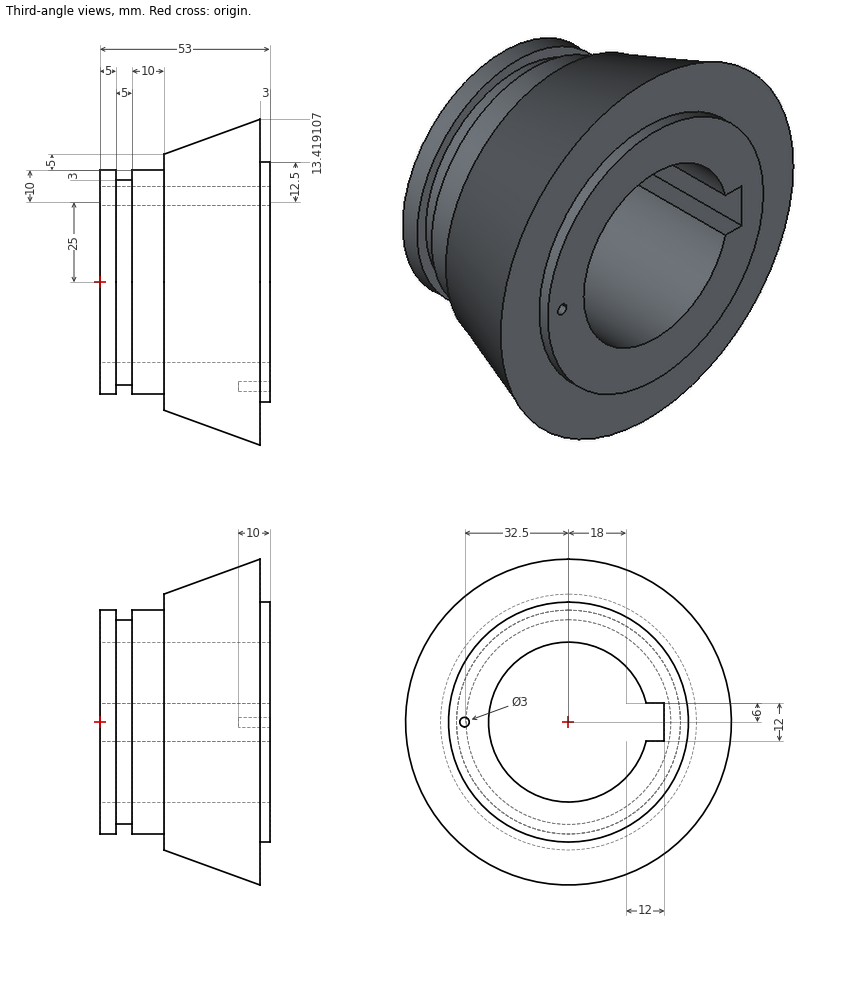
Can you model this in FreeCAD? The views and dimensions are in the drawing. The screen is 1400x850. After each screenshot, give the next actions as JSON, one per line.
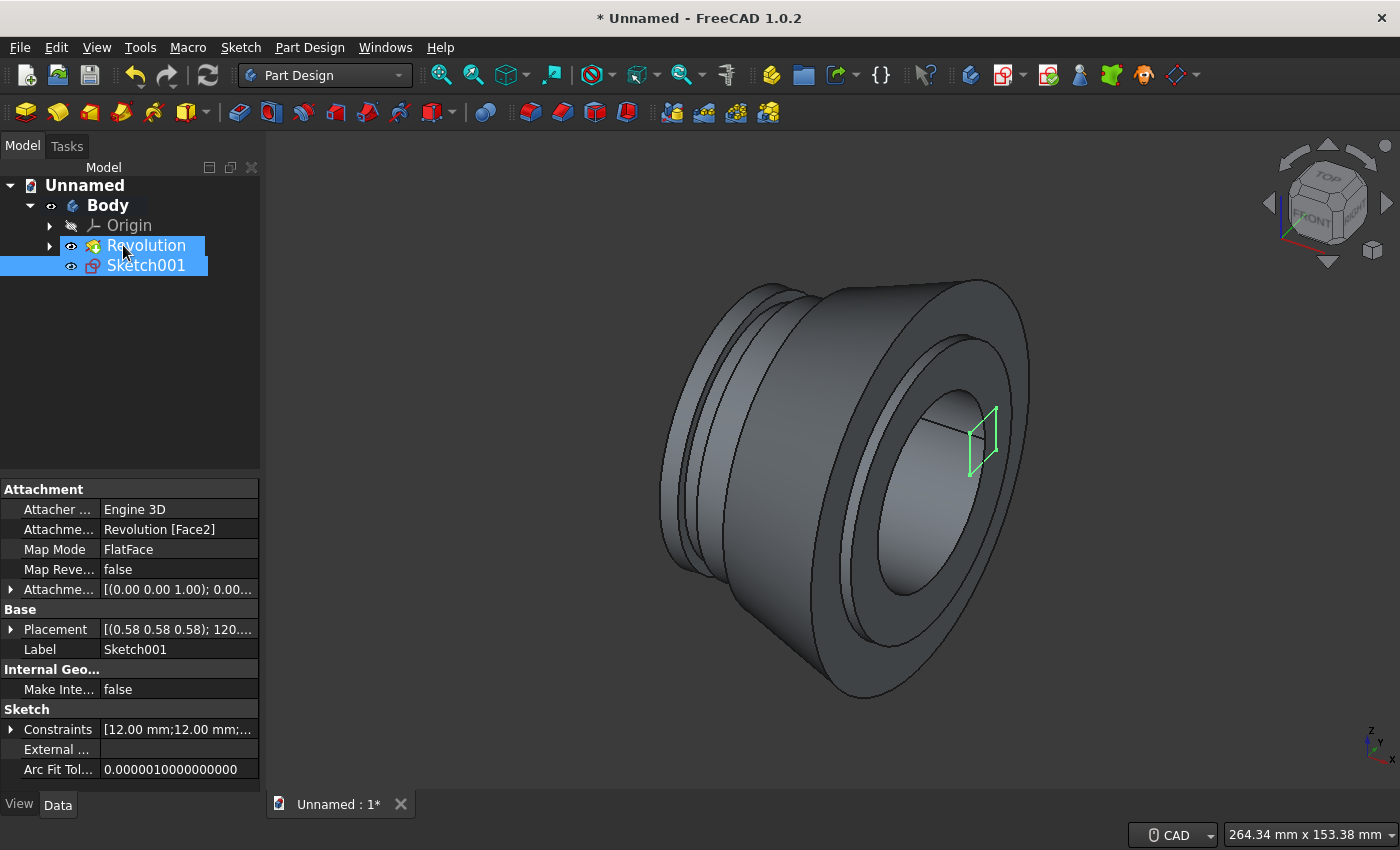
{"action": "left_click", "coordinate": [240, 112]}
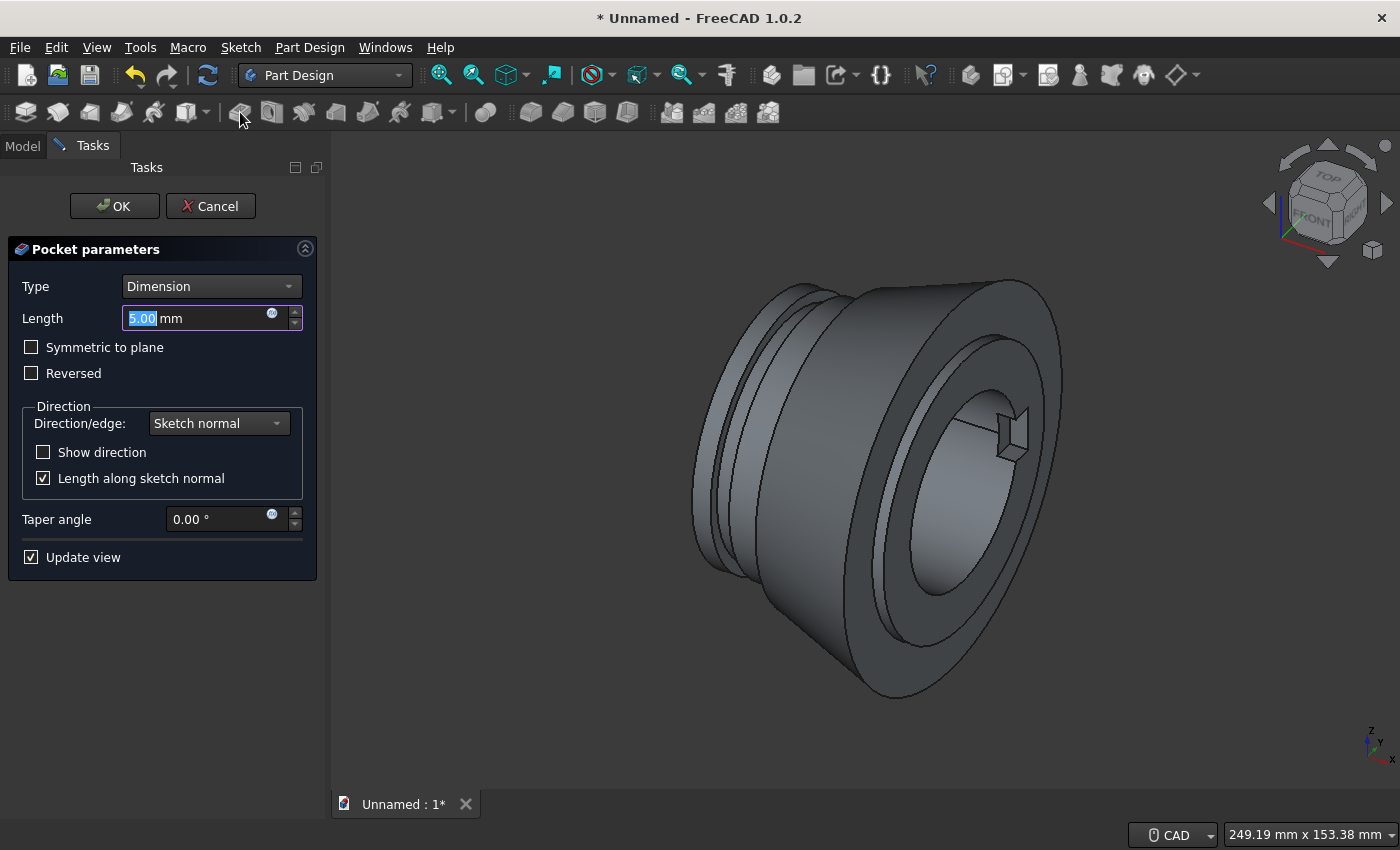
{"action": "left_click", "coordinate": [212, 286]}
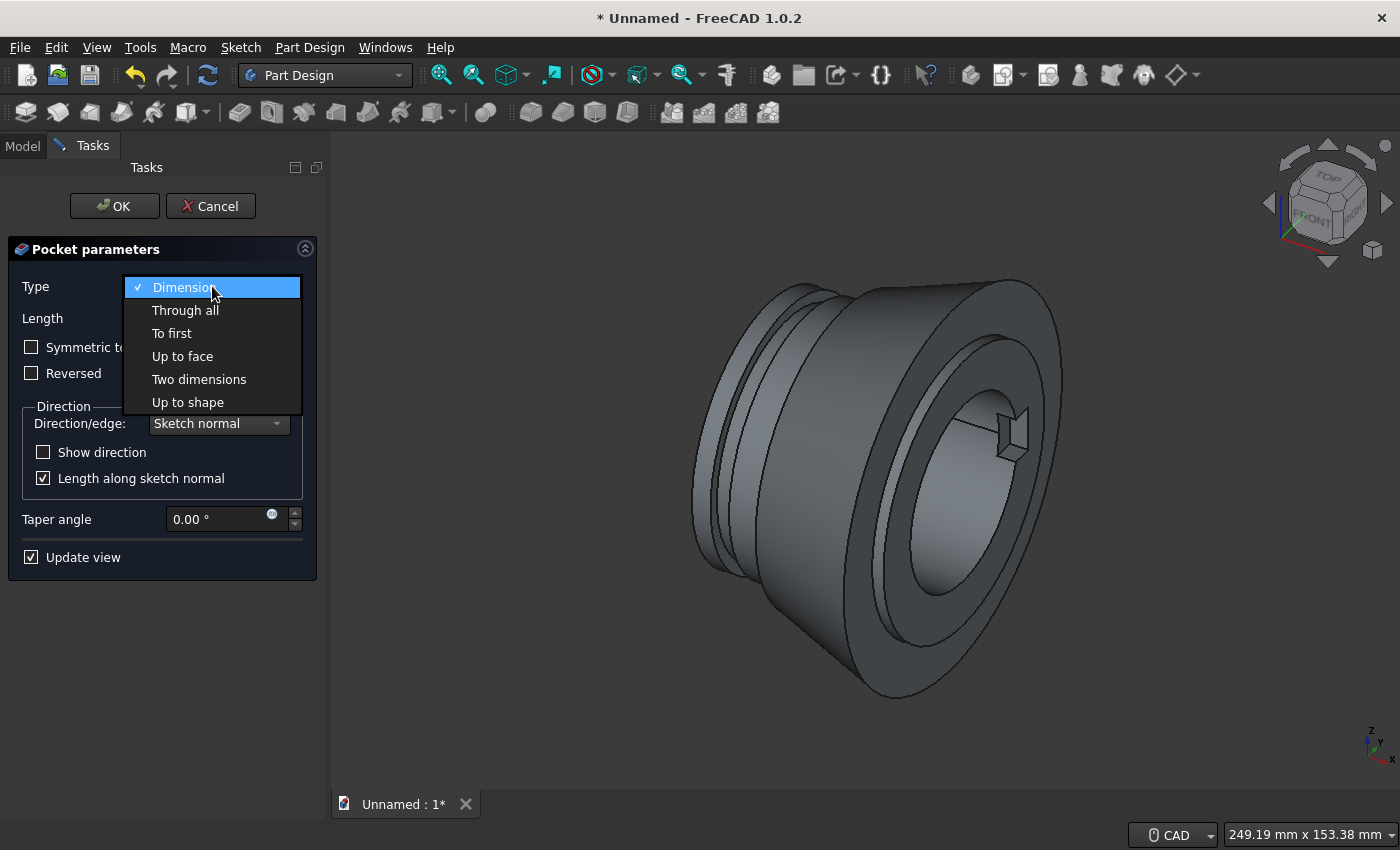
{"action": "left_click", "coordinate": [212, 310]}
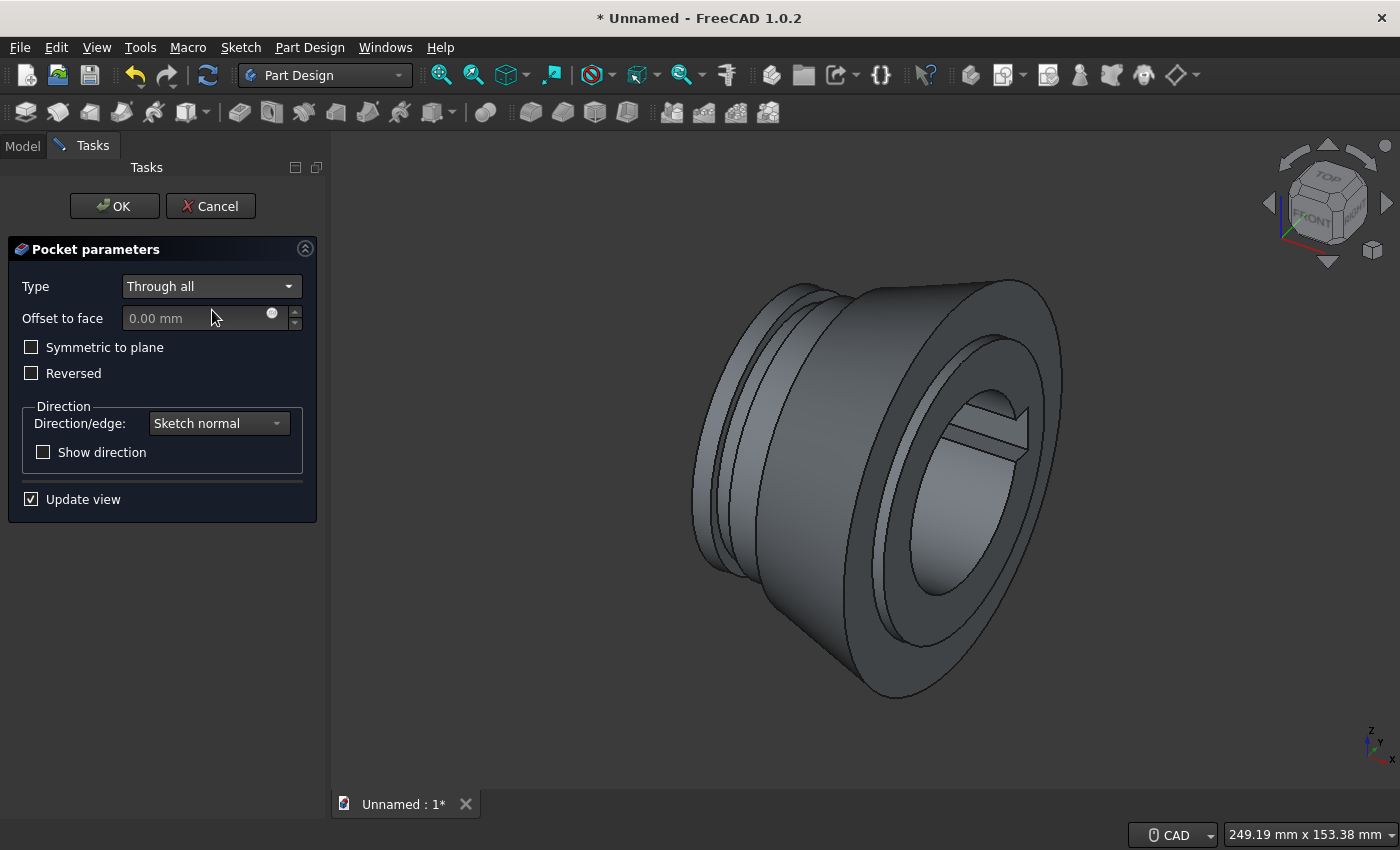
{"action": "left_click", "coordinate": [115, 206]}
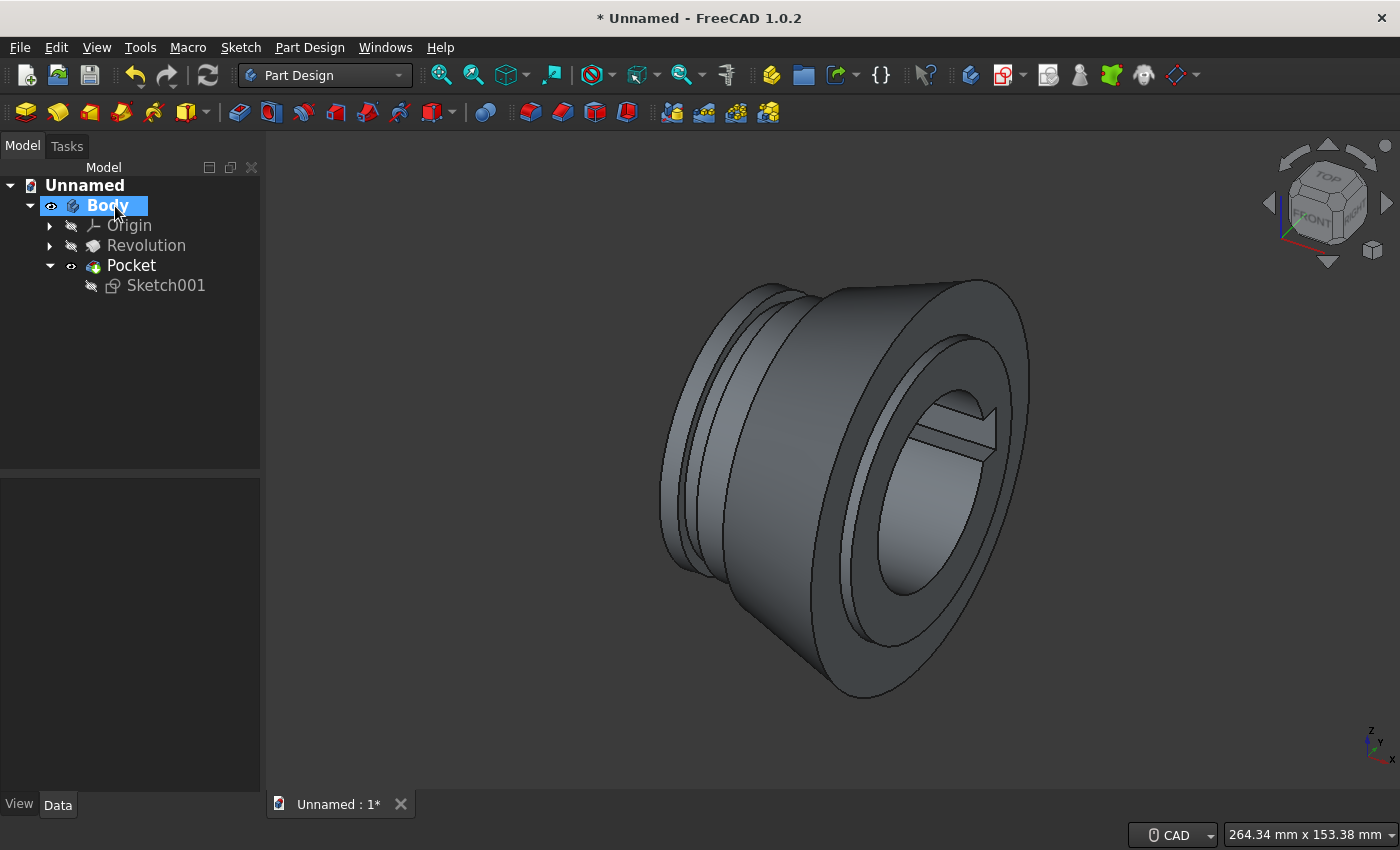
{"action": "left_click", "coordinate": [931, 379]}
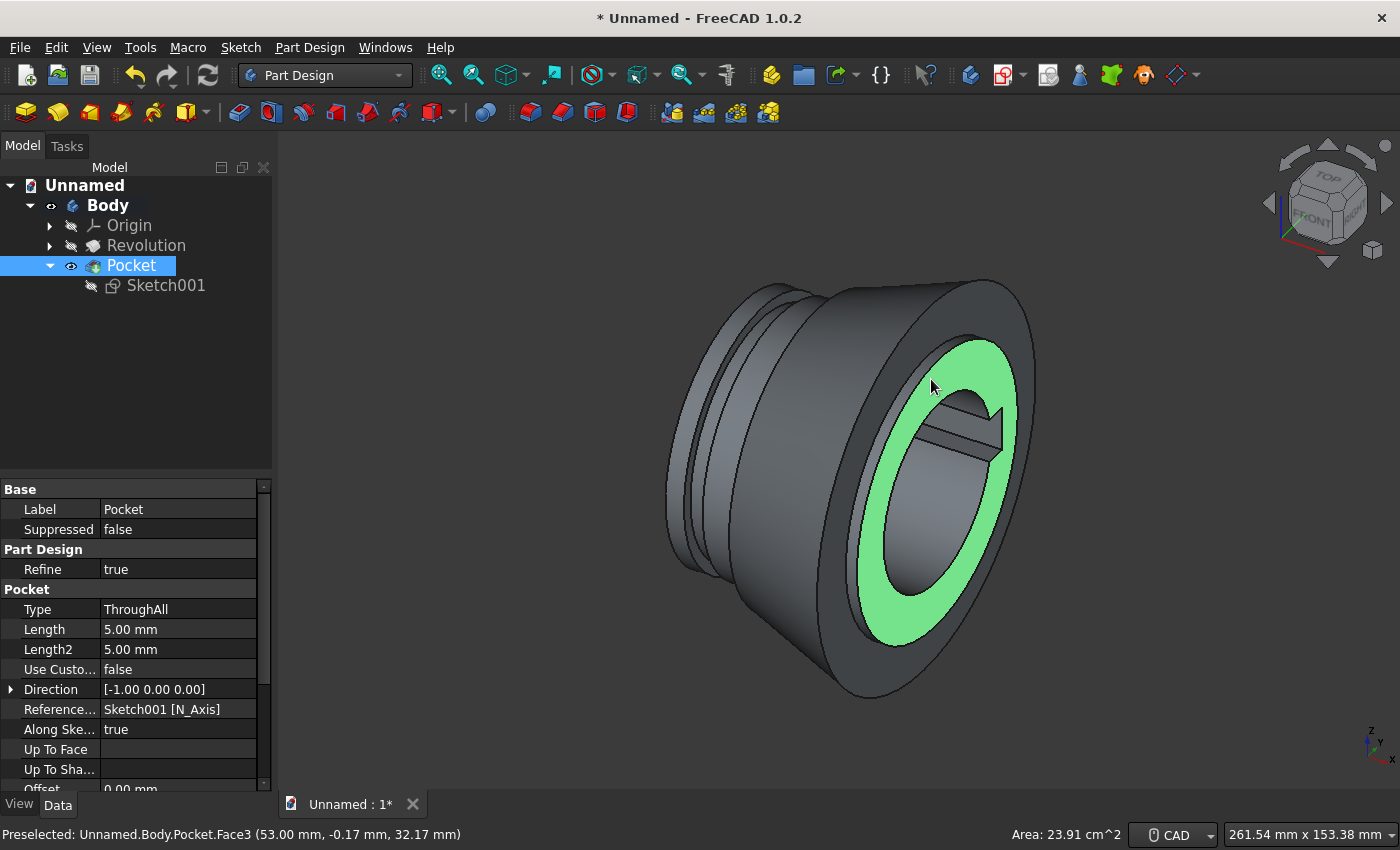
{"action": "left_click", "coordinate": [1004, 76]}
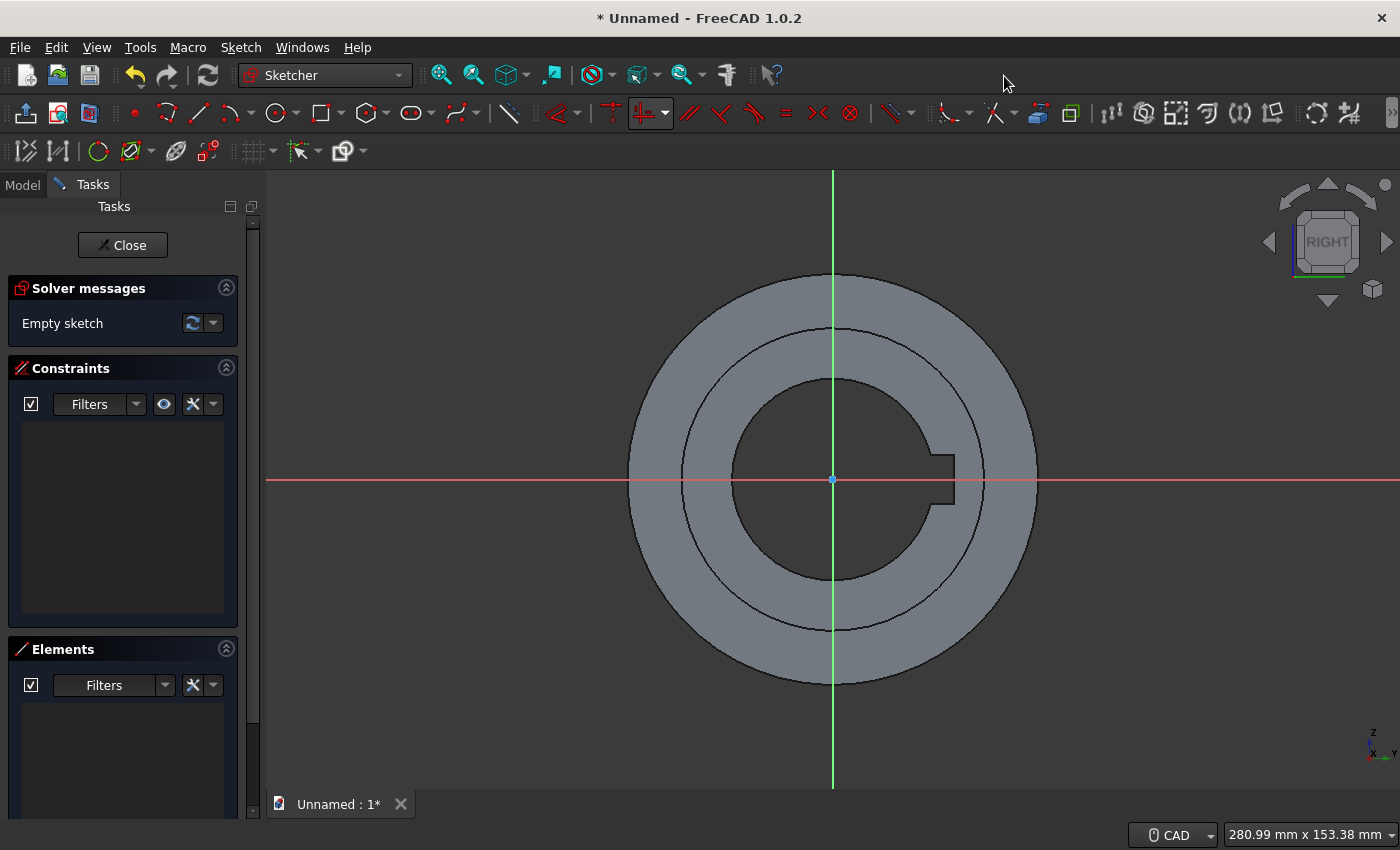
{"action": "scroll", "coordinate": [698, 479], "scroll_direction": "up", "scroll_amount": 15}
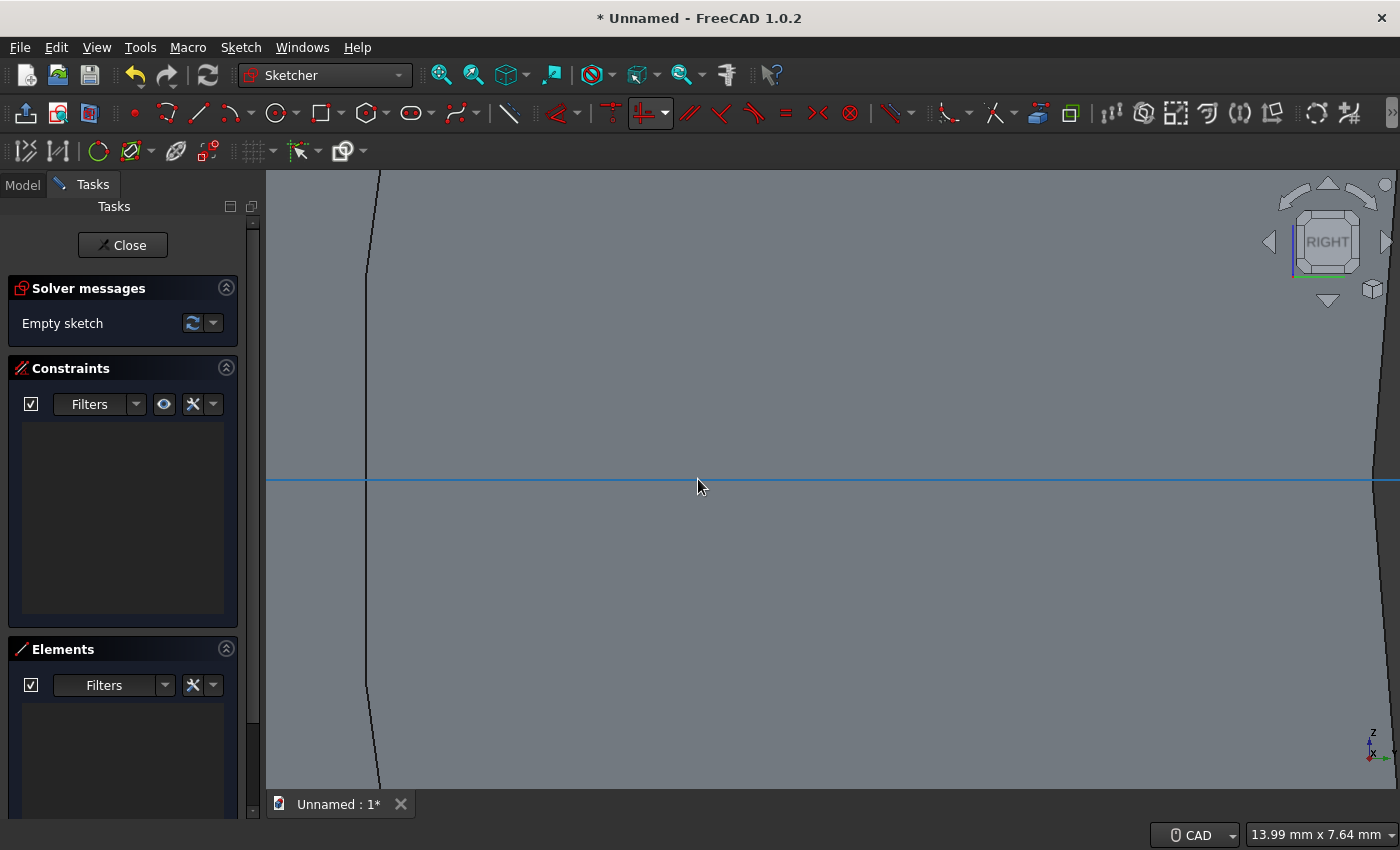
{"action": "scroll", "coordinate": [764, 480], "scroll_direction": "up", "scroll_amount": 2}